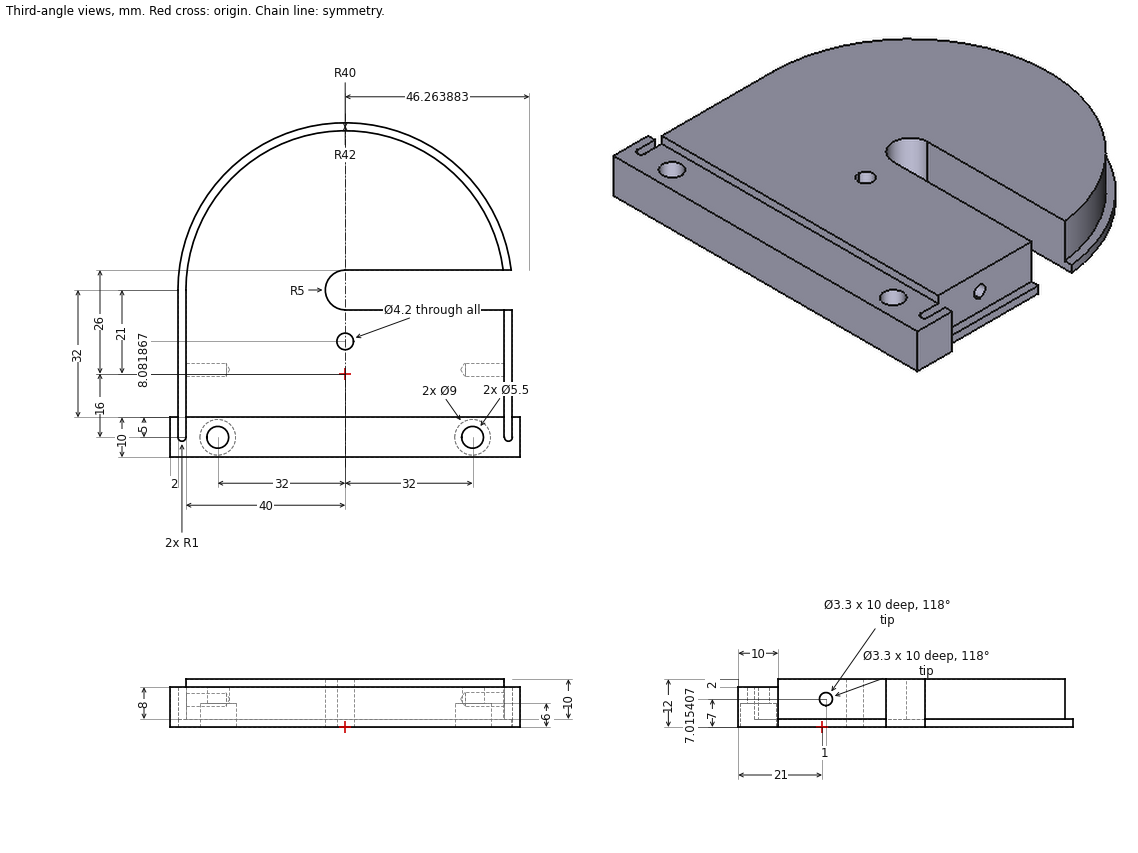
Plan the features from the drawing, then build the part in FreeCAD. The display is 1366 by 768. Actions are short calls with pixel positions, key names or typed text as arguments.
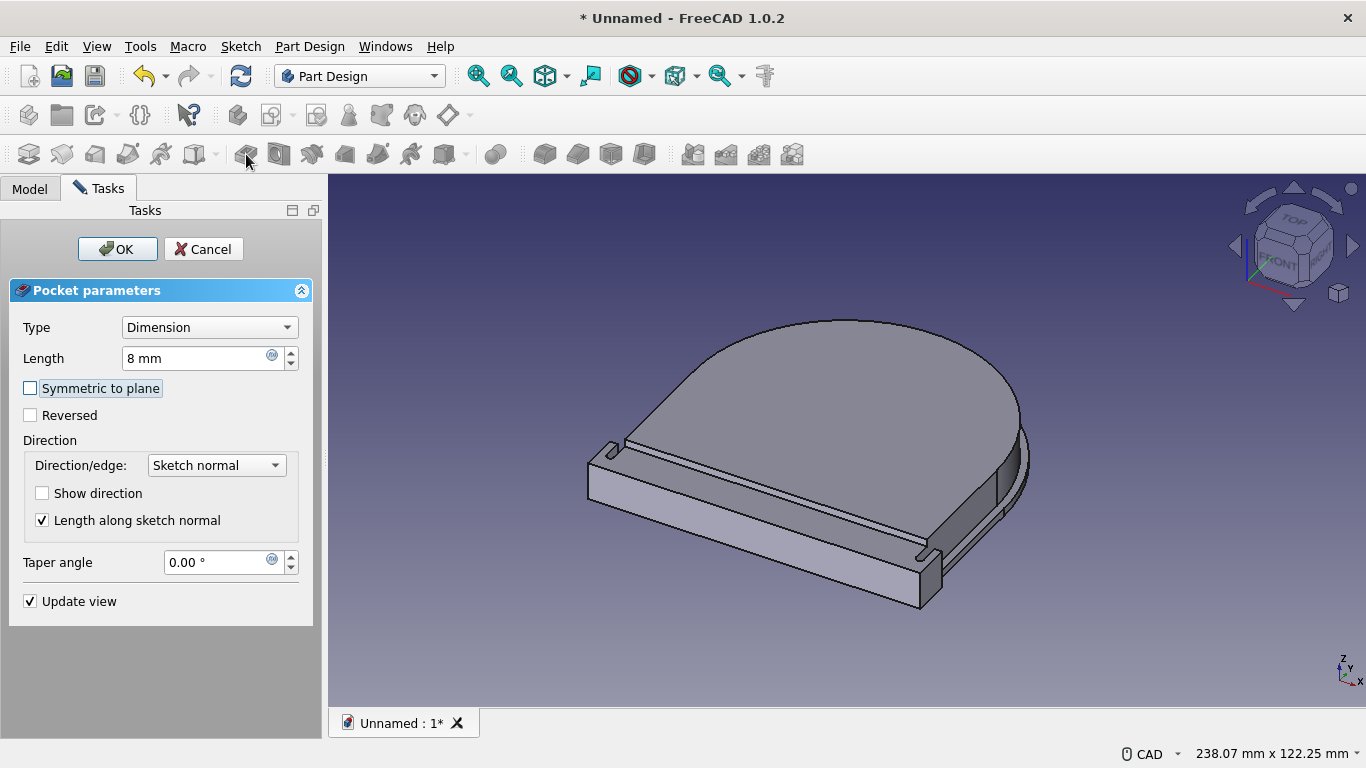
click(118, 249)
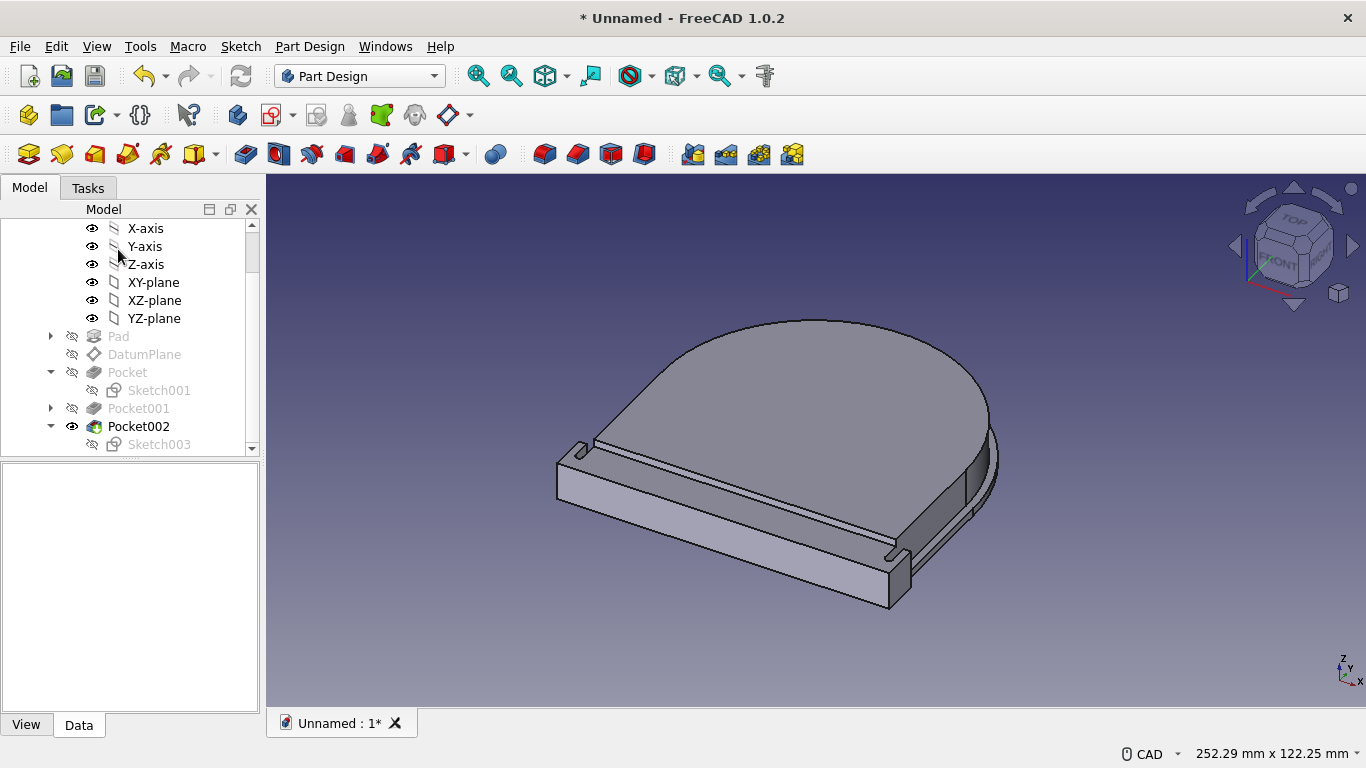
click(270, 116)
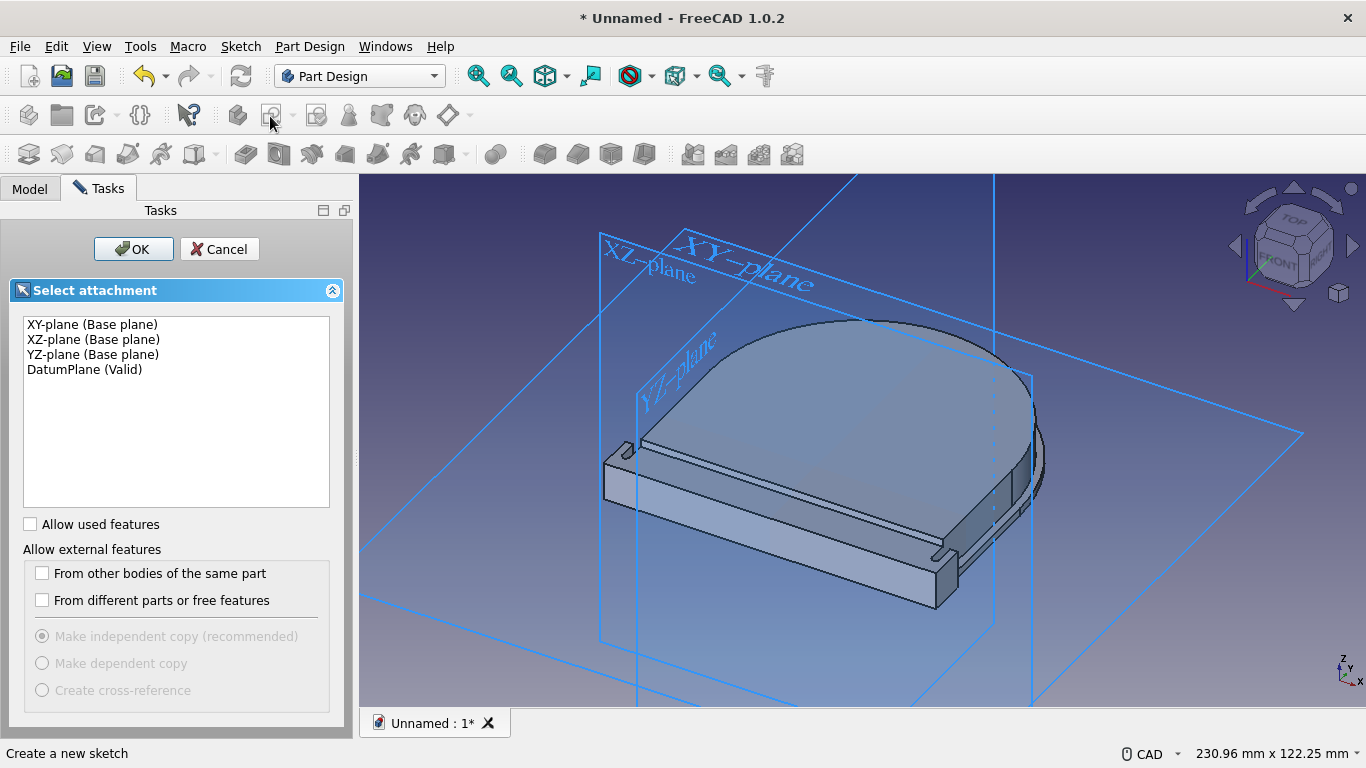
click(84, 324)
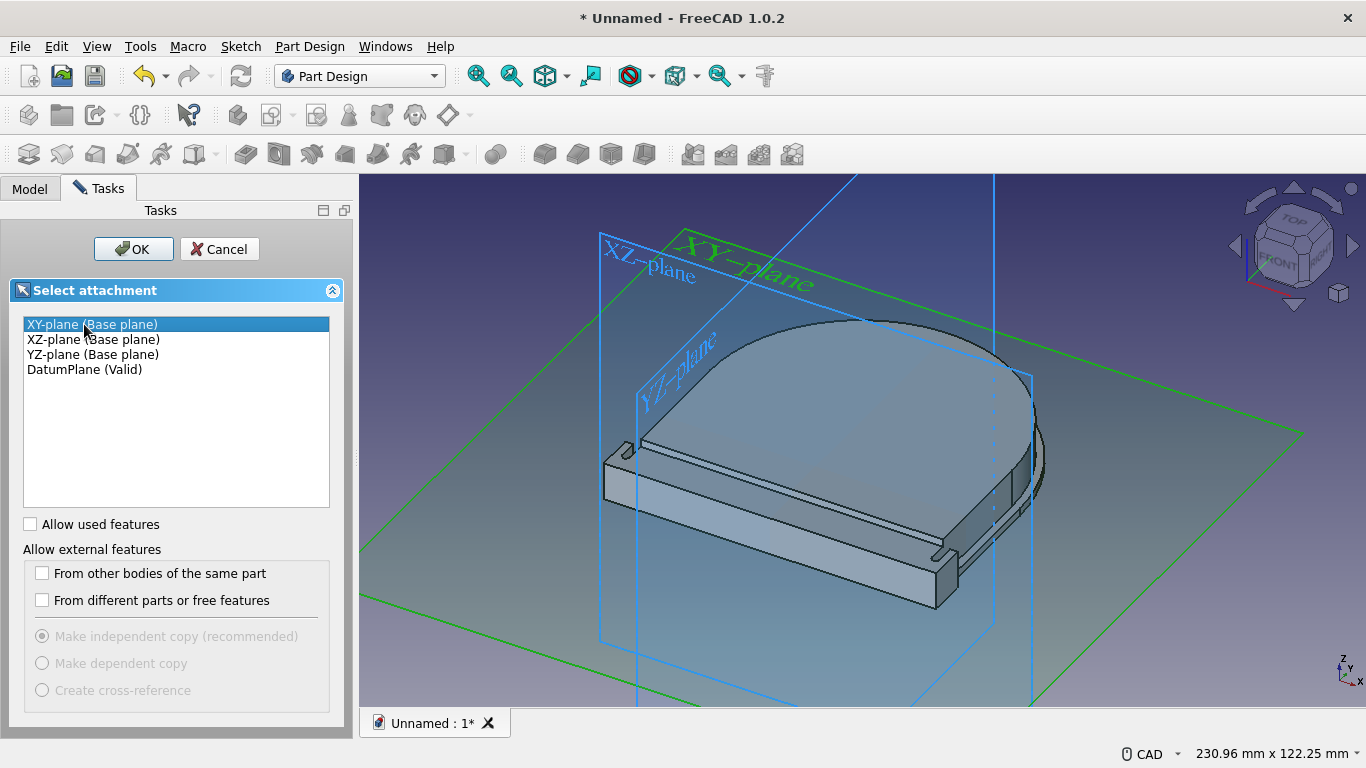
click(134, 249)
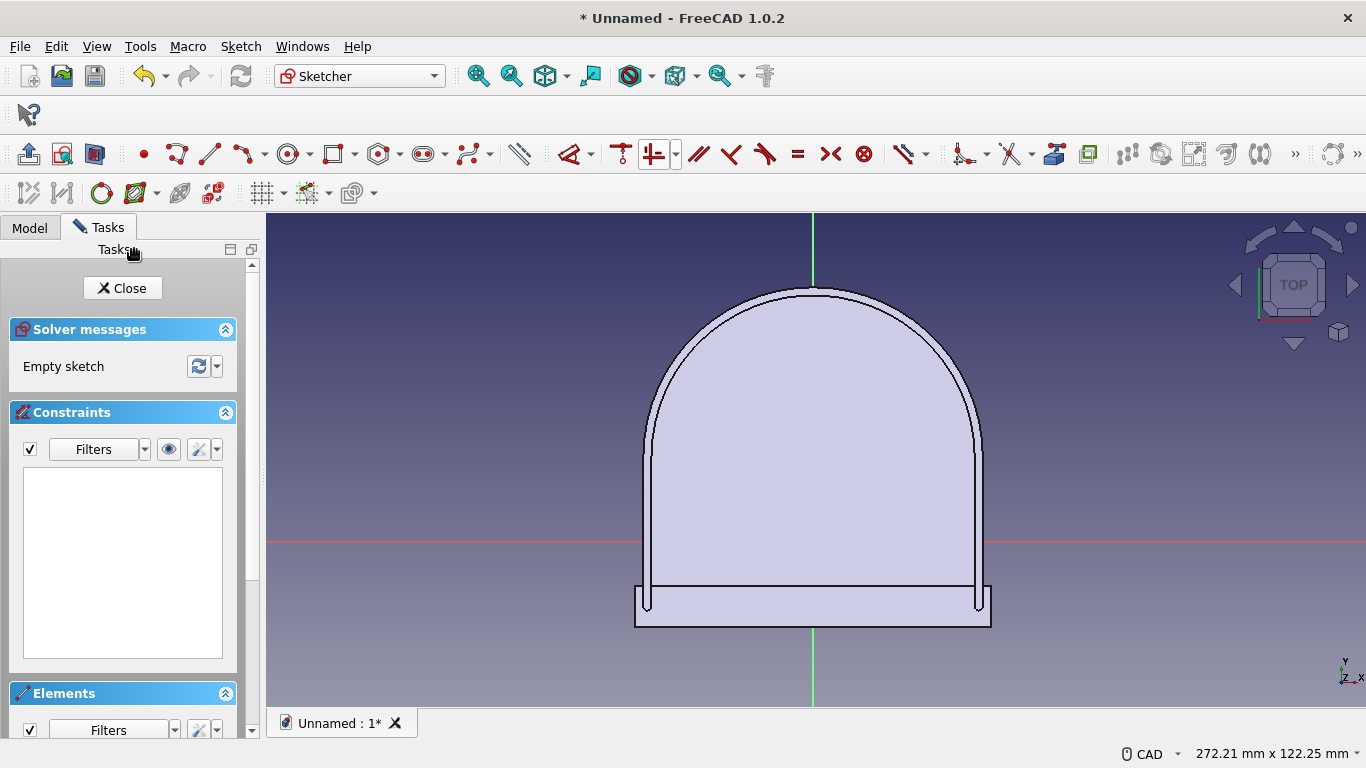
click(95, 154)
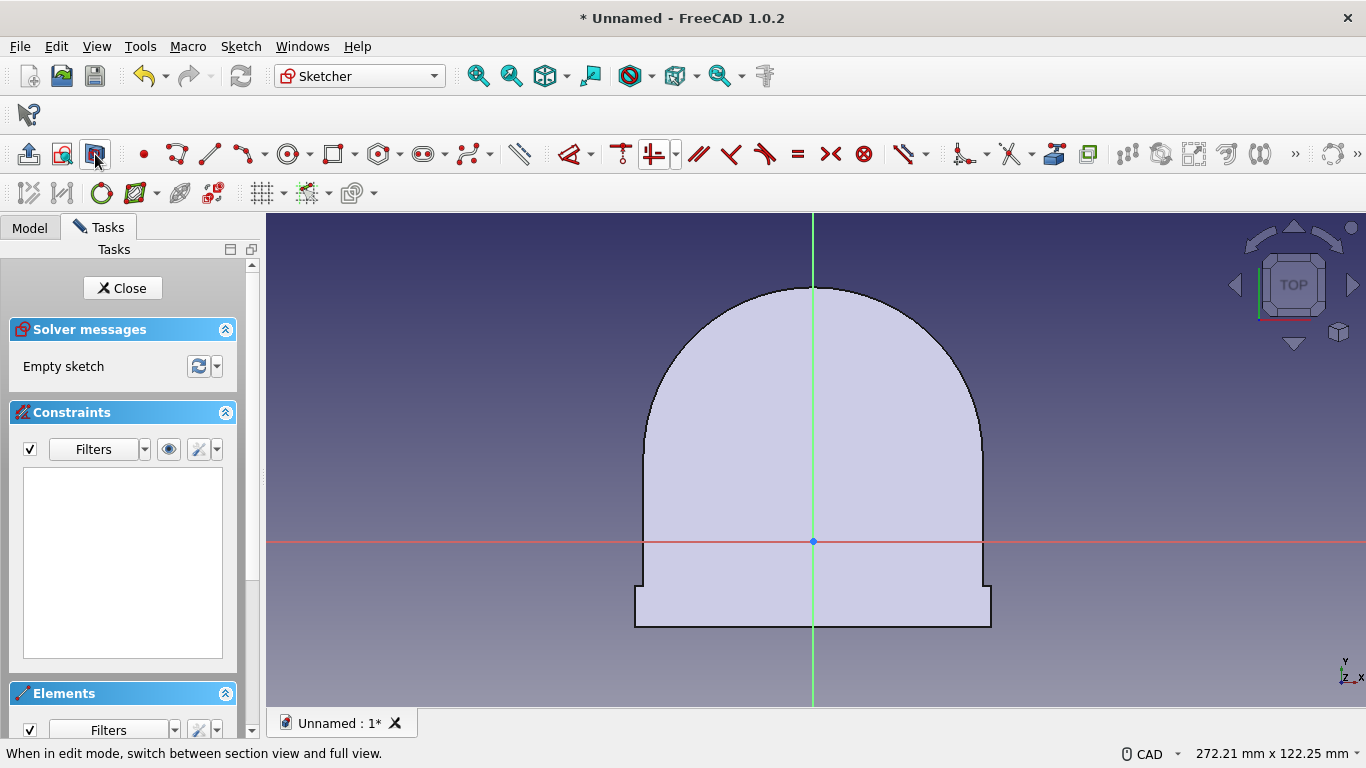
scroll(983, 506, up, 5)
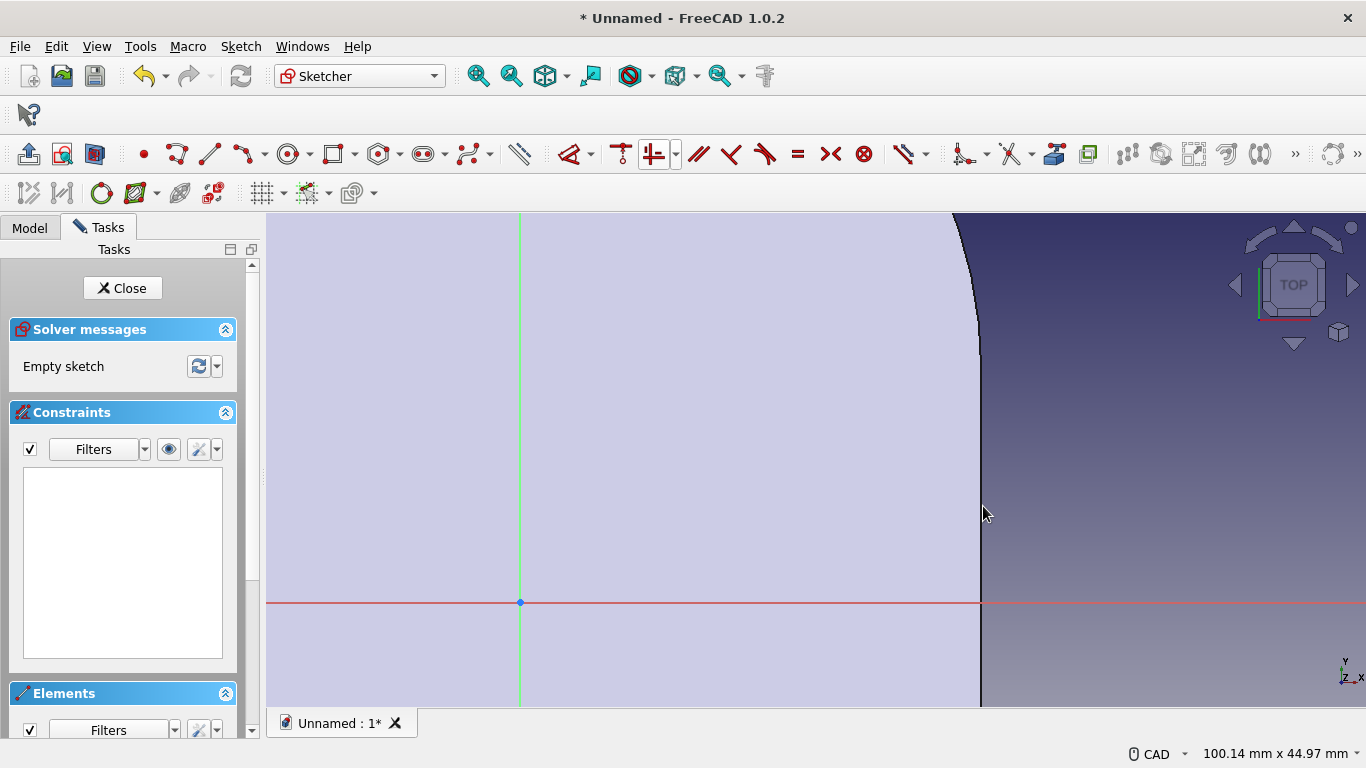
click(177, 154)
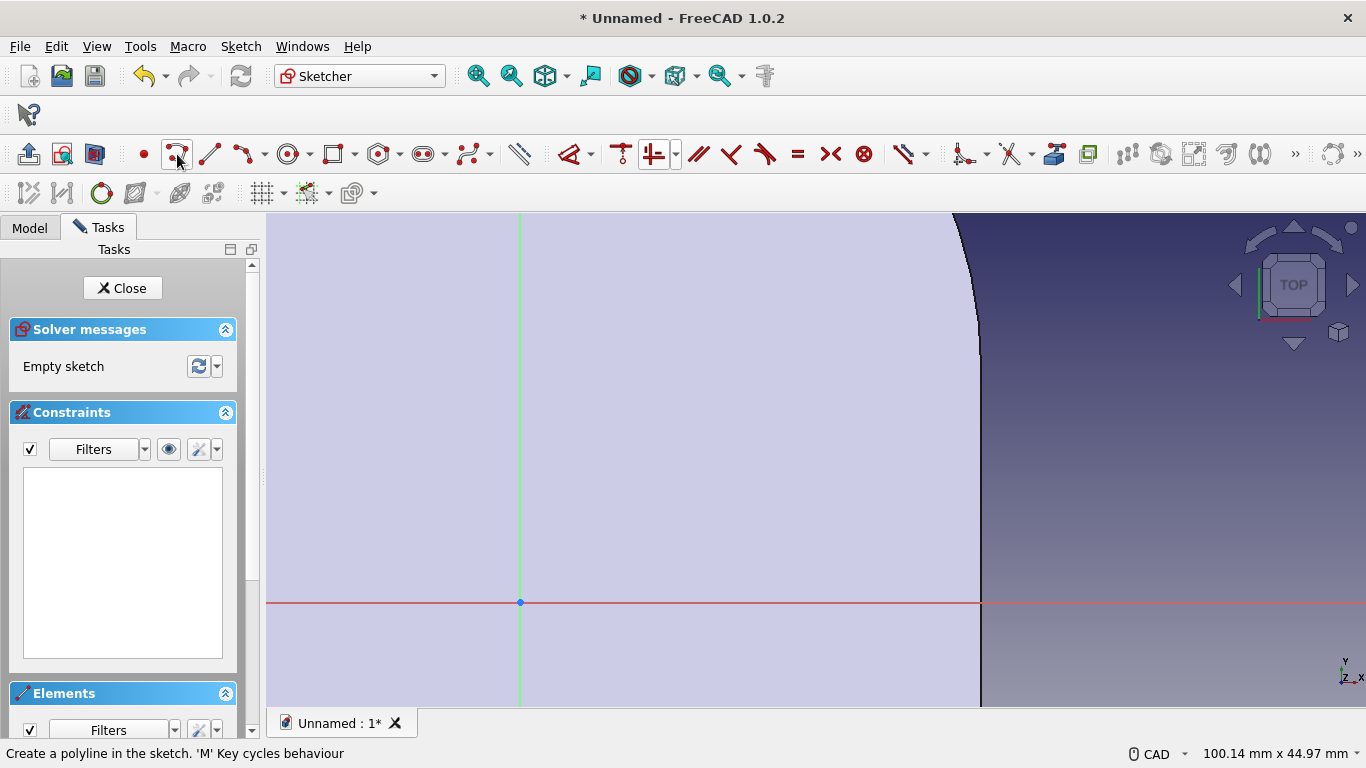
click(520, 317)
click(1028, 317)
click(1028, 427)
click(520, 427)
right_click(520, 427)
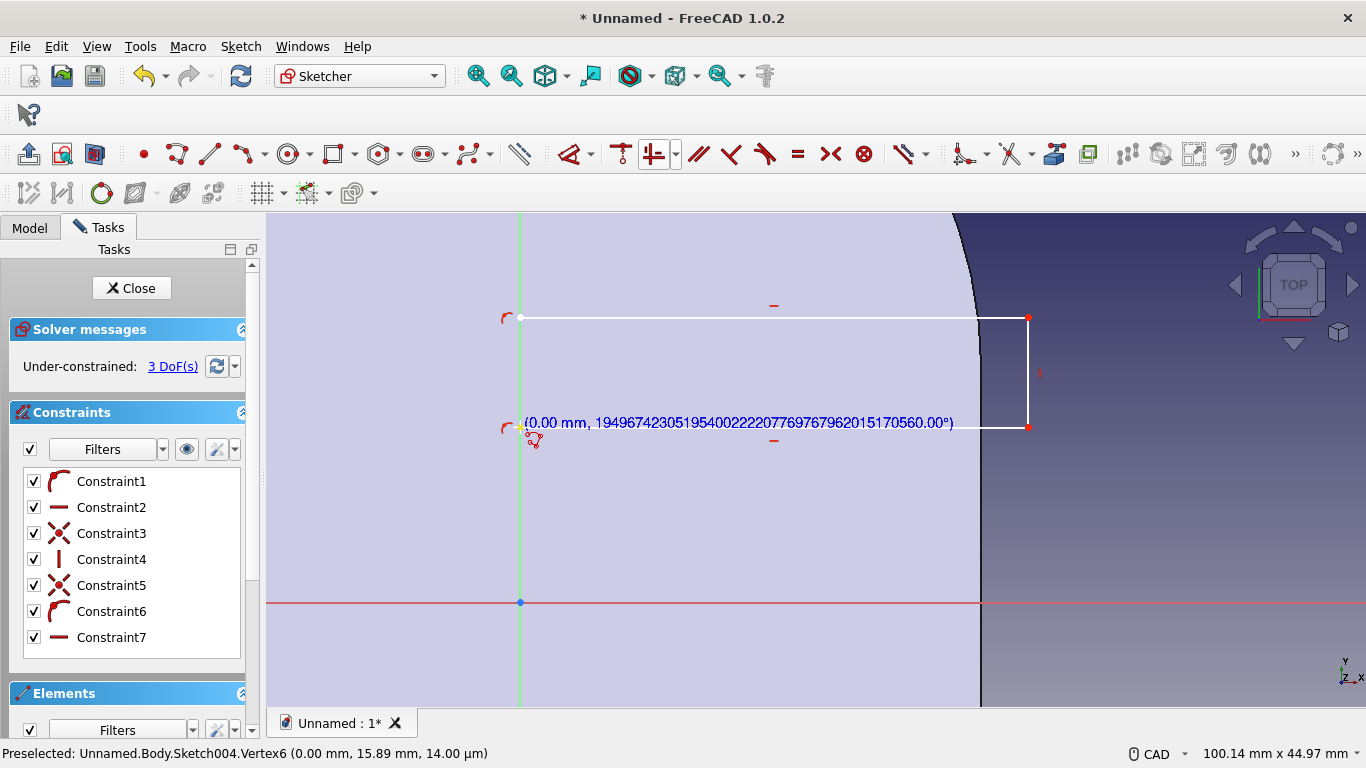
click(242, 154)